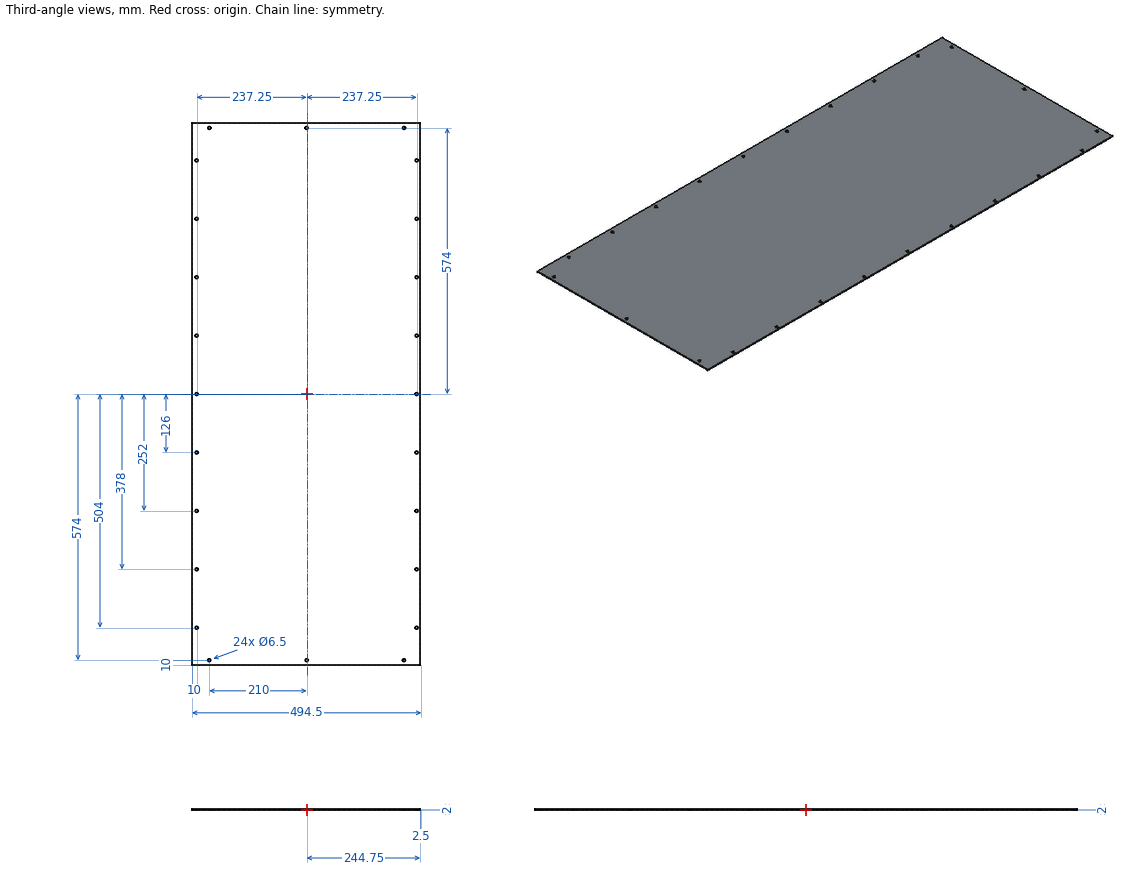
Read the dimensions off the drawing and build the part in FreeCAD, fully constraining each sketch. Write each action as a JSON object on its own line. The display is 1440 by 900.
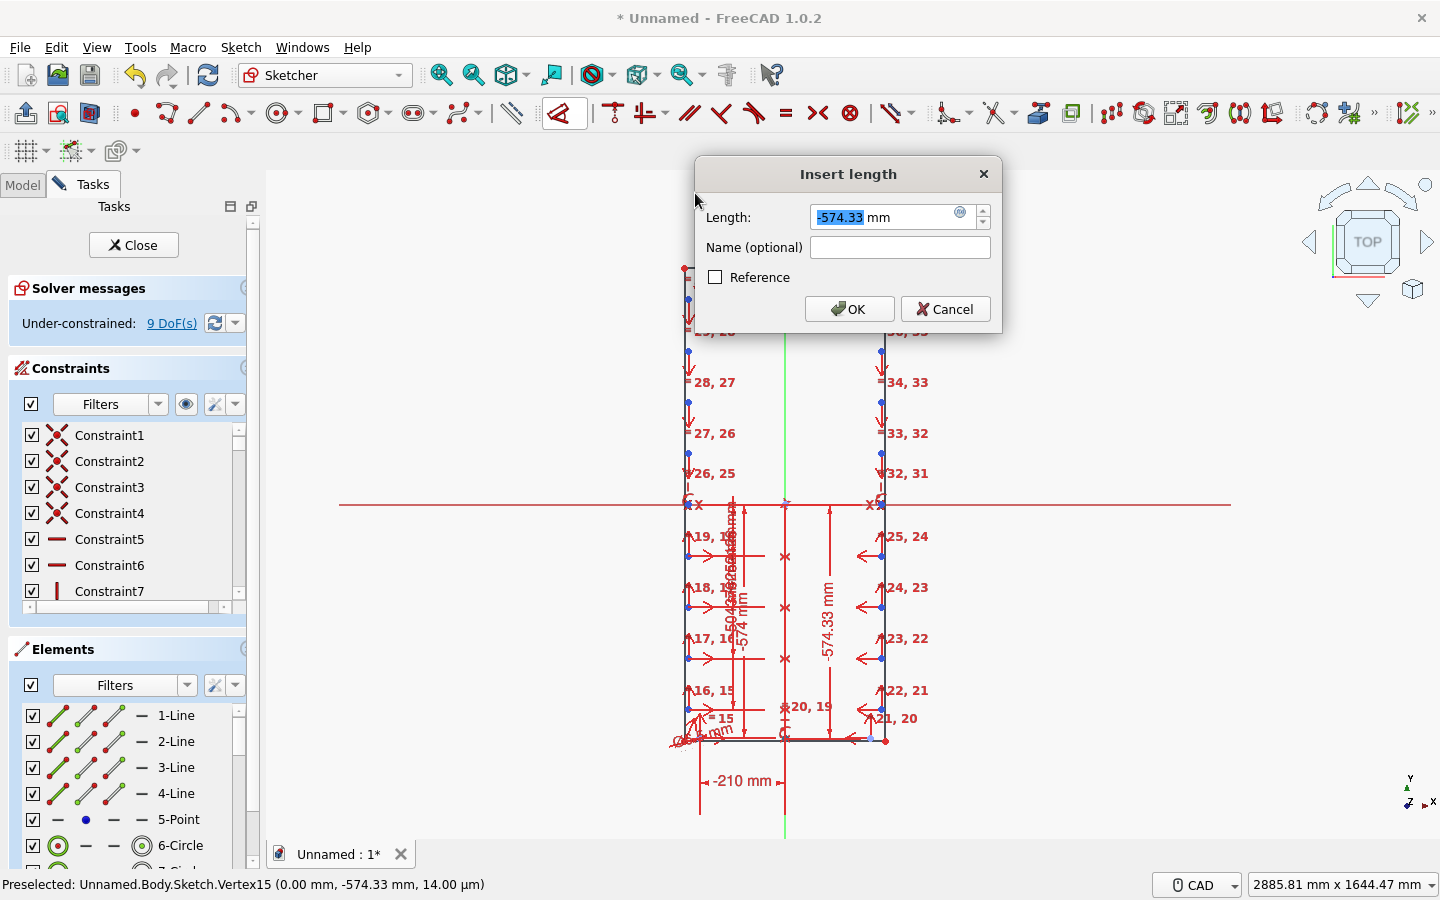
{"action": "type", "text": "-574"}
{"action": "key", "text": "Return"}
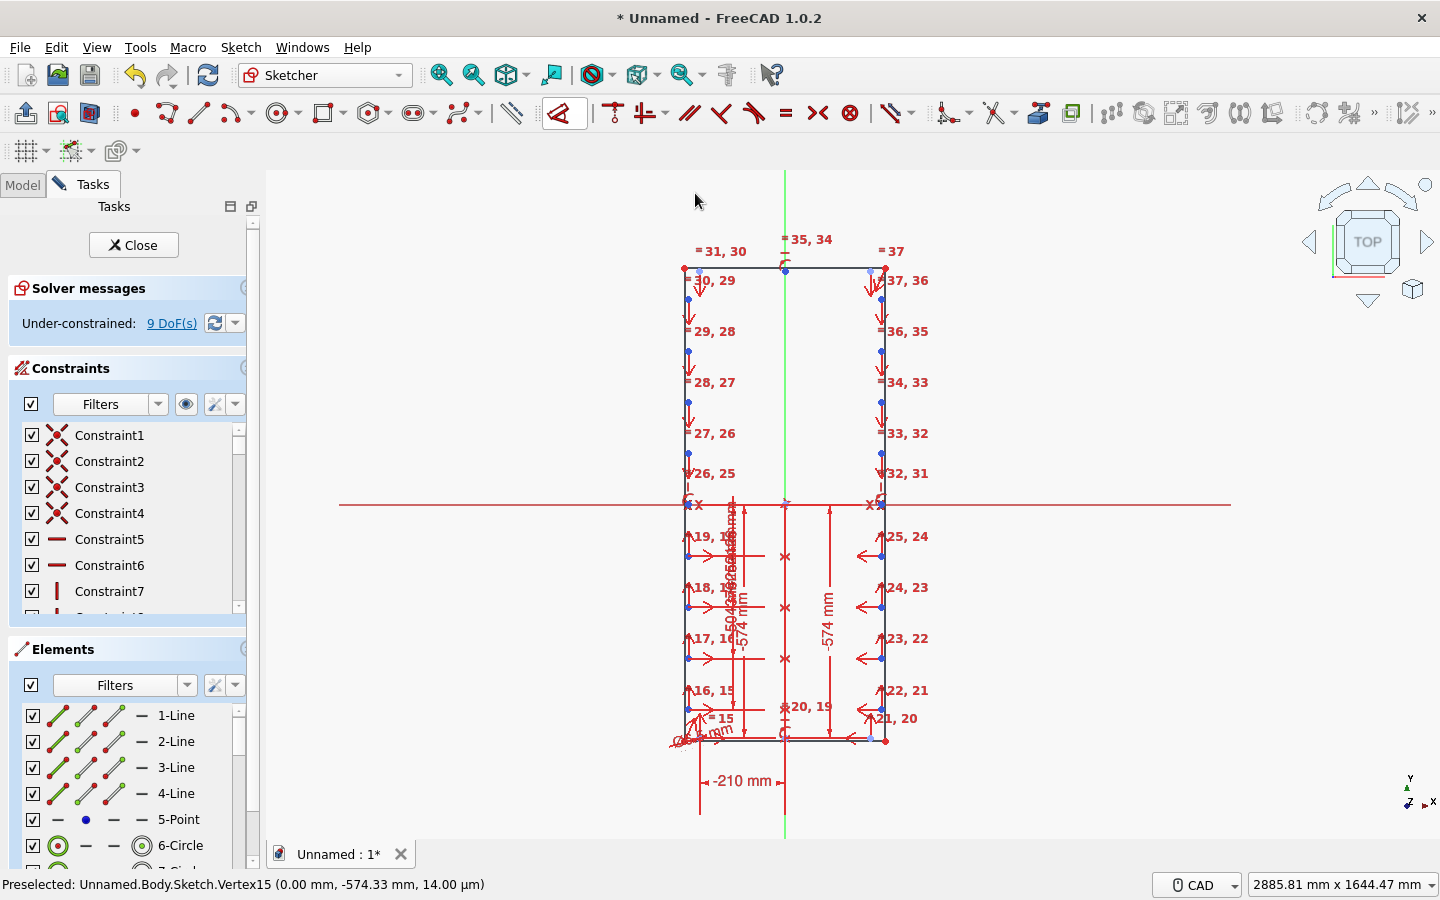
{"action": "left_click", "coordinate": [785, 272]}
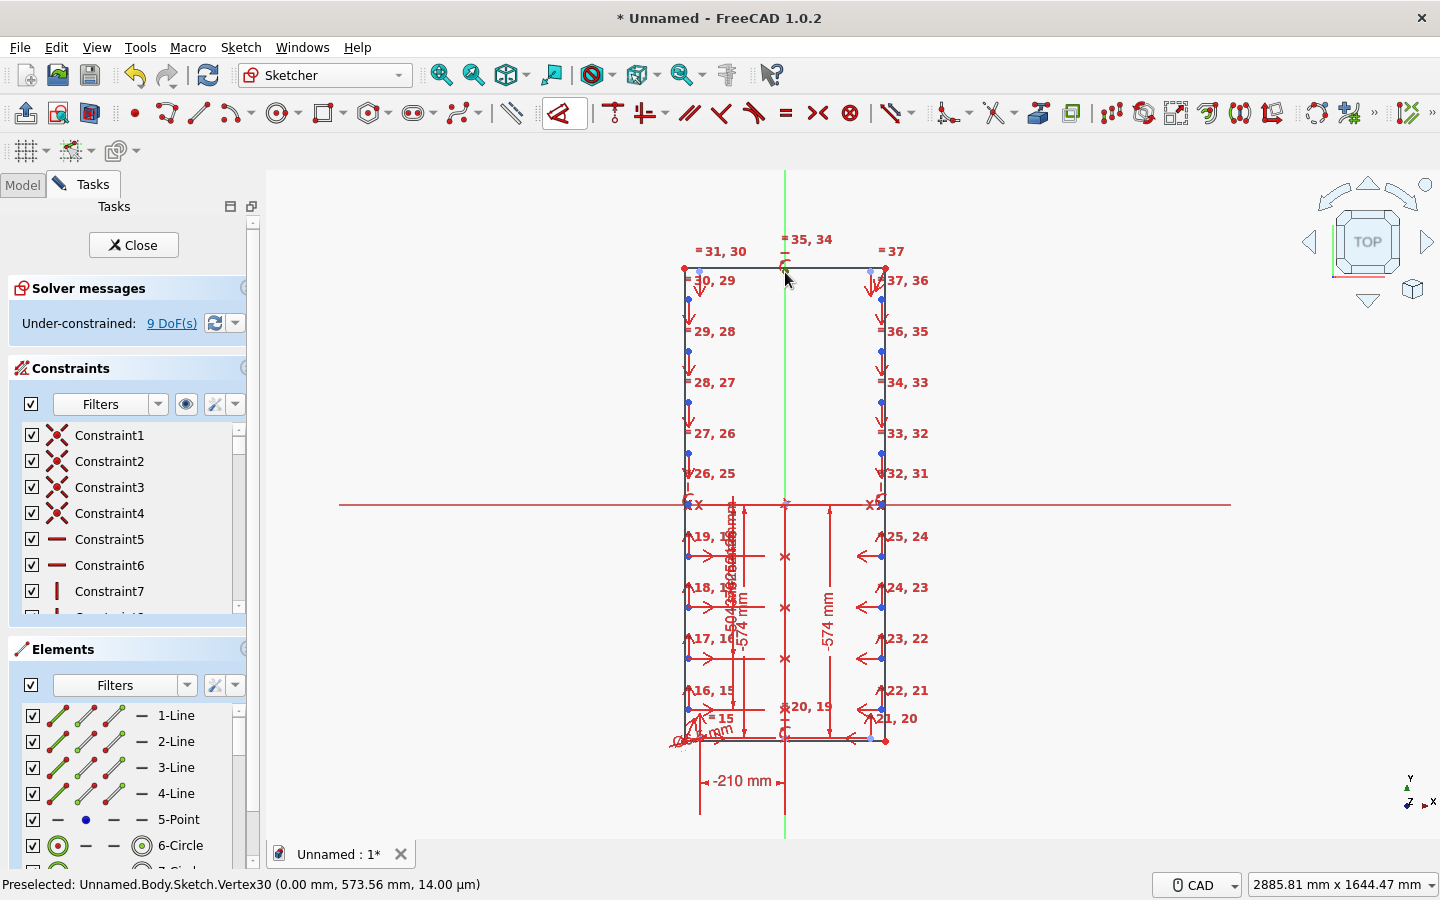
{"action": "key", "text": "i"}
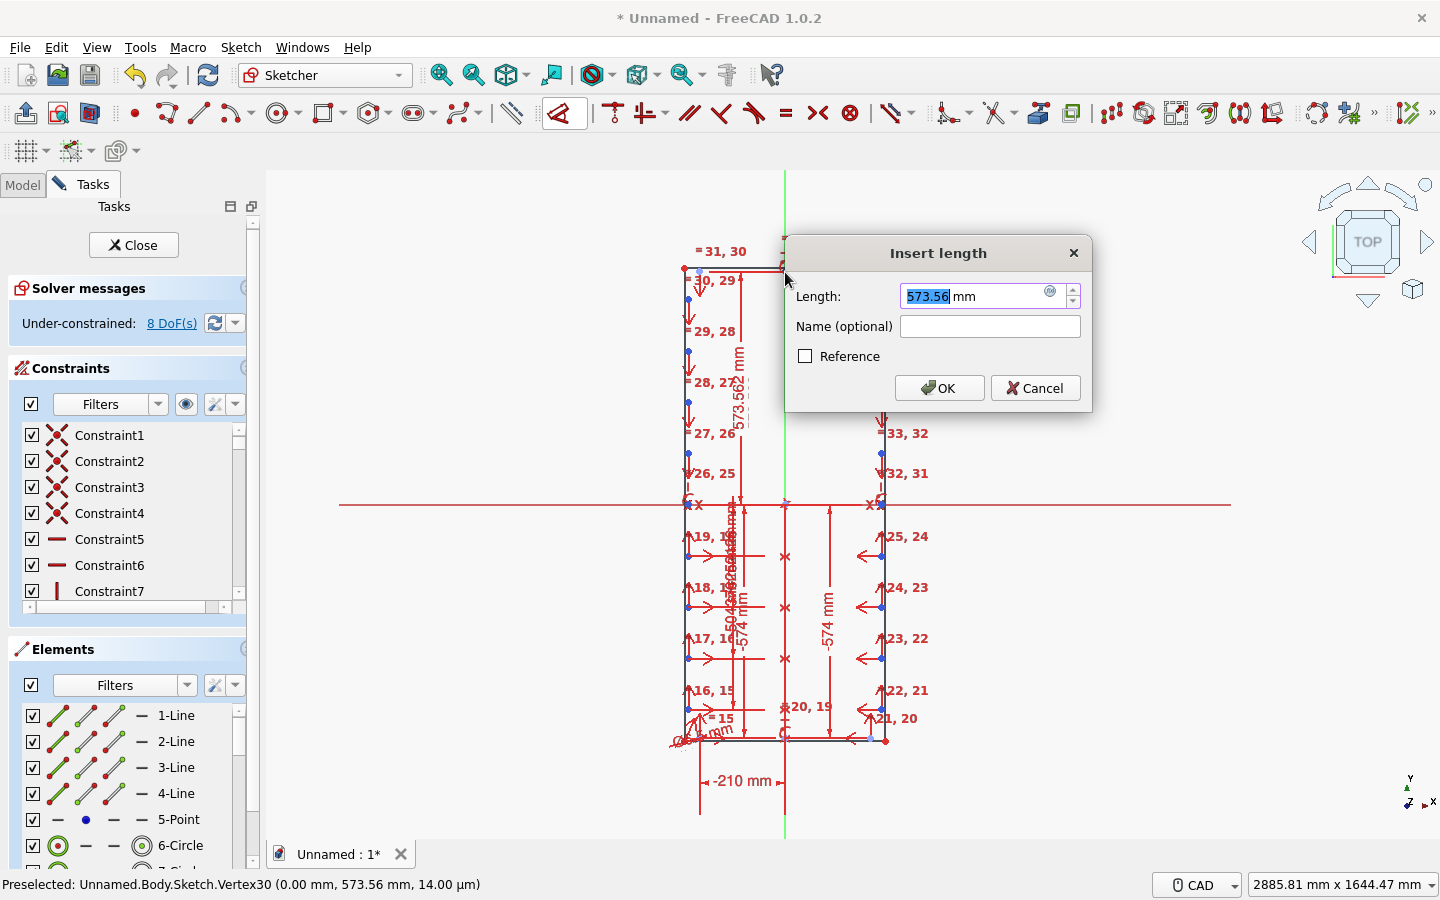
{"action": "type", "text": "574"}
{"action": "key", "text": "Return"}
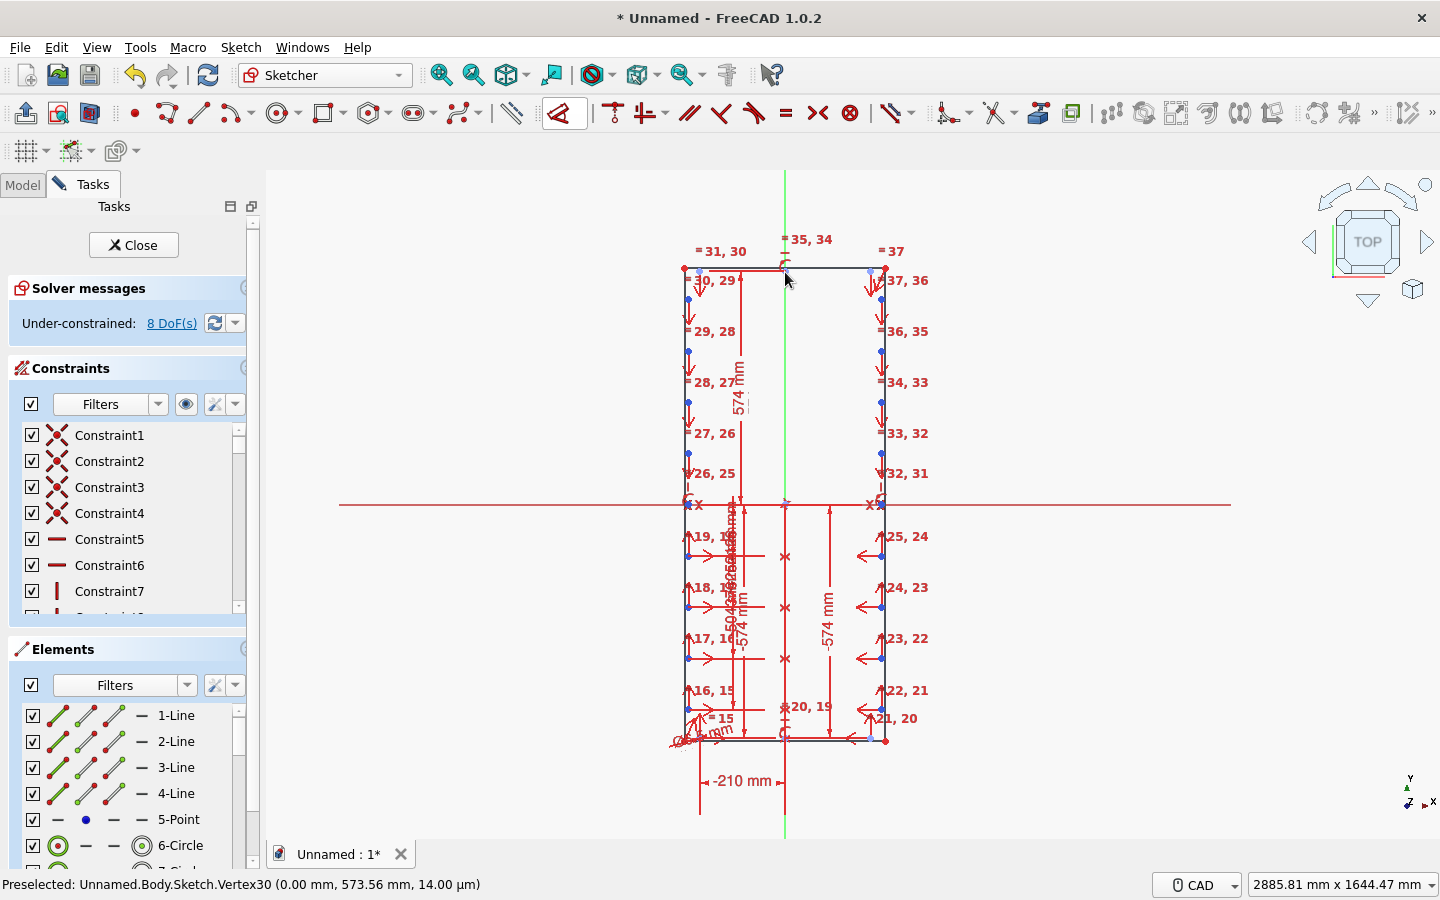
{"action": "scroll", "coordinate": [685, 741], "scroll_direction": "up", "scroll_amount": 12}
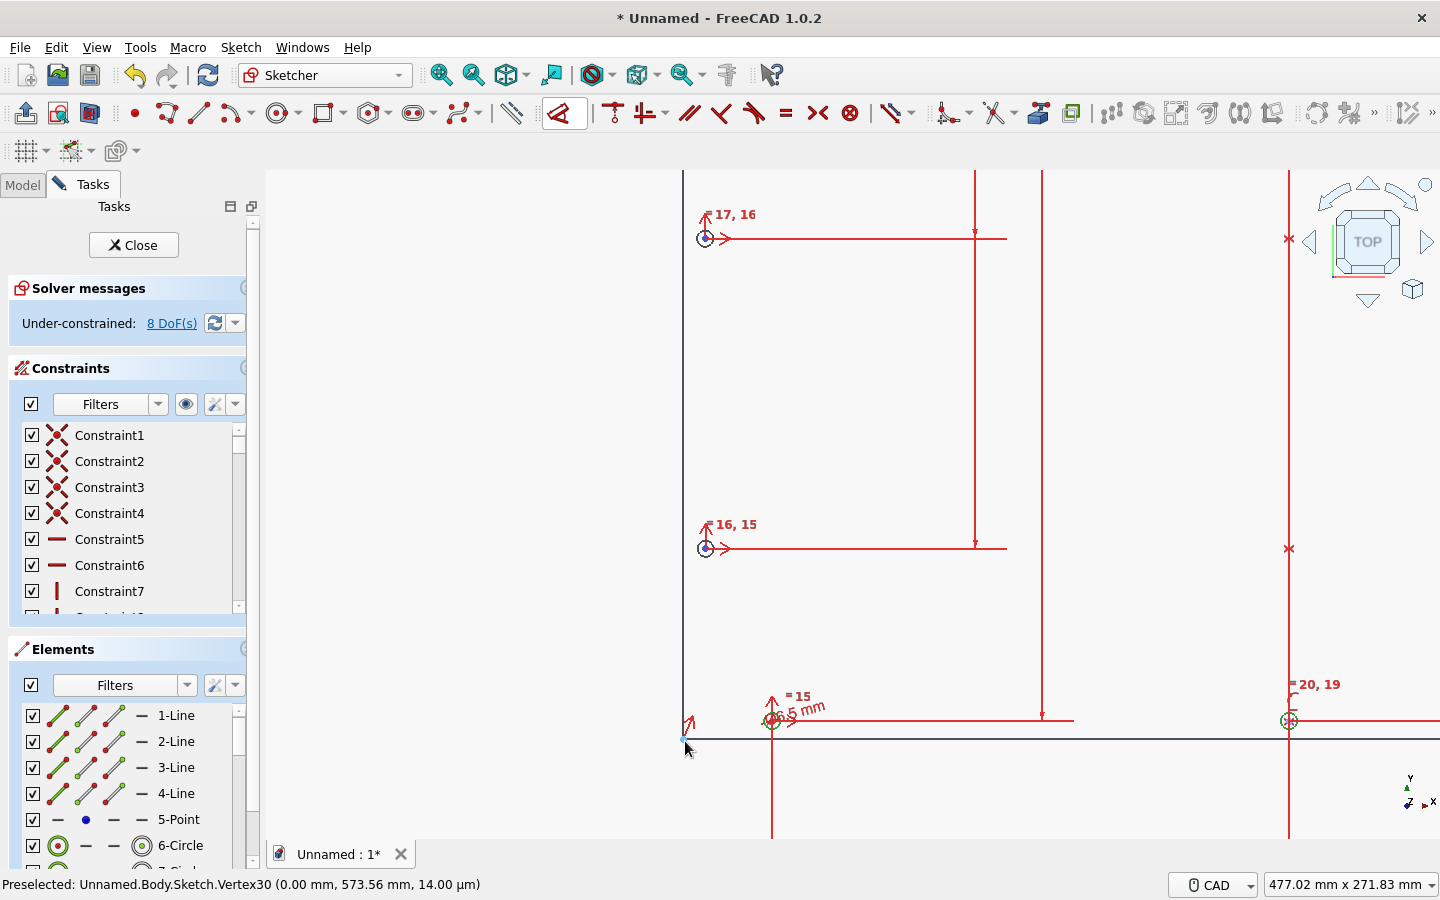
{"action": "left_click", "coordinate": [681, 737]}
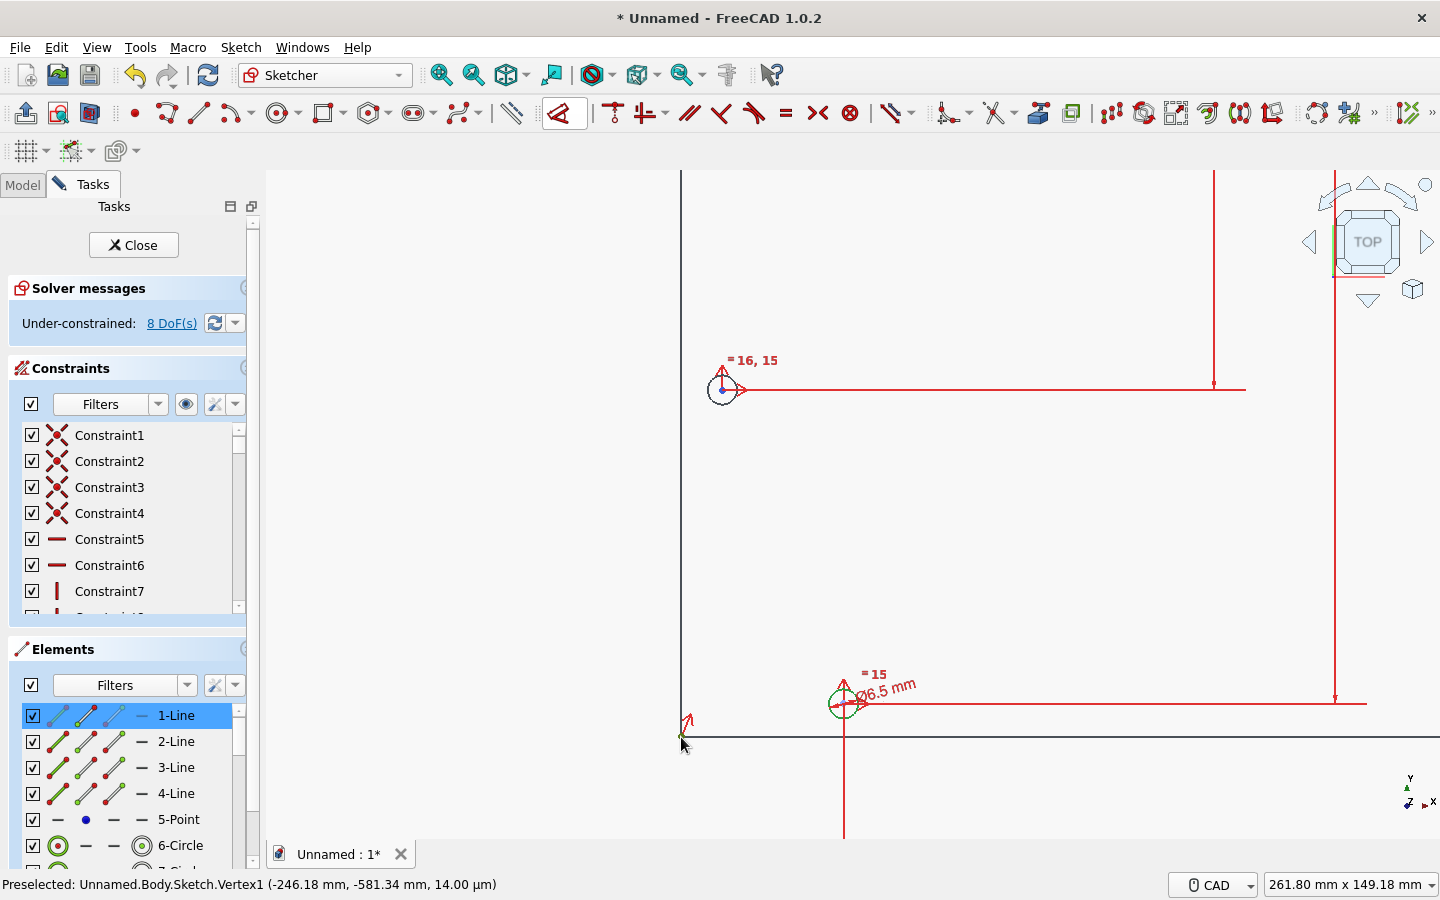
{"action": "left_click", "coordinate": [844, 704]}